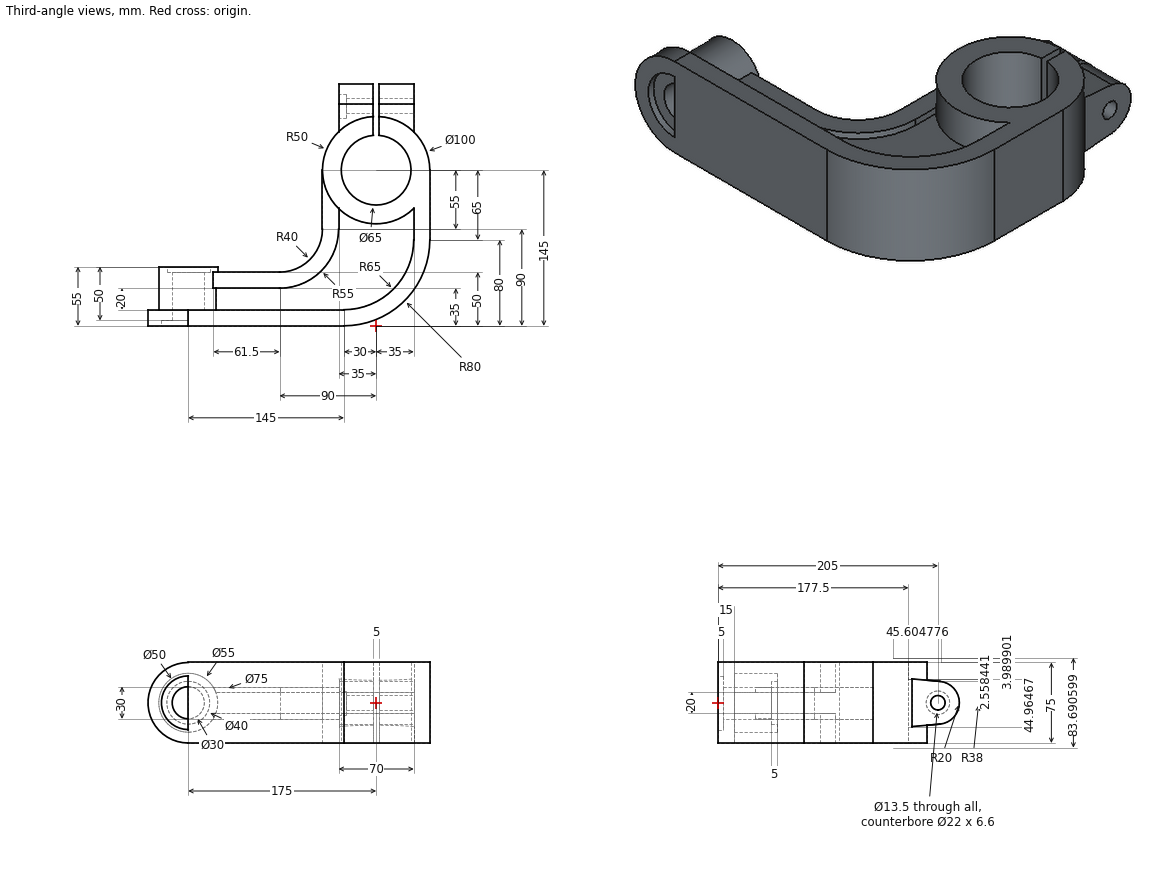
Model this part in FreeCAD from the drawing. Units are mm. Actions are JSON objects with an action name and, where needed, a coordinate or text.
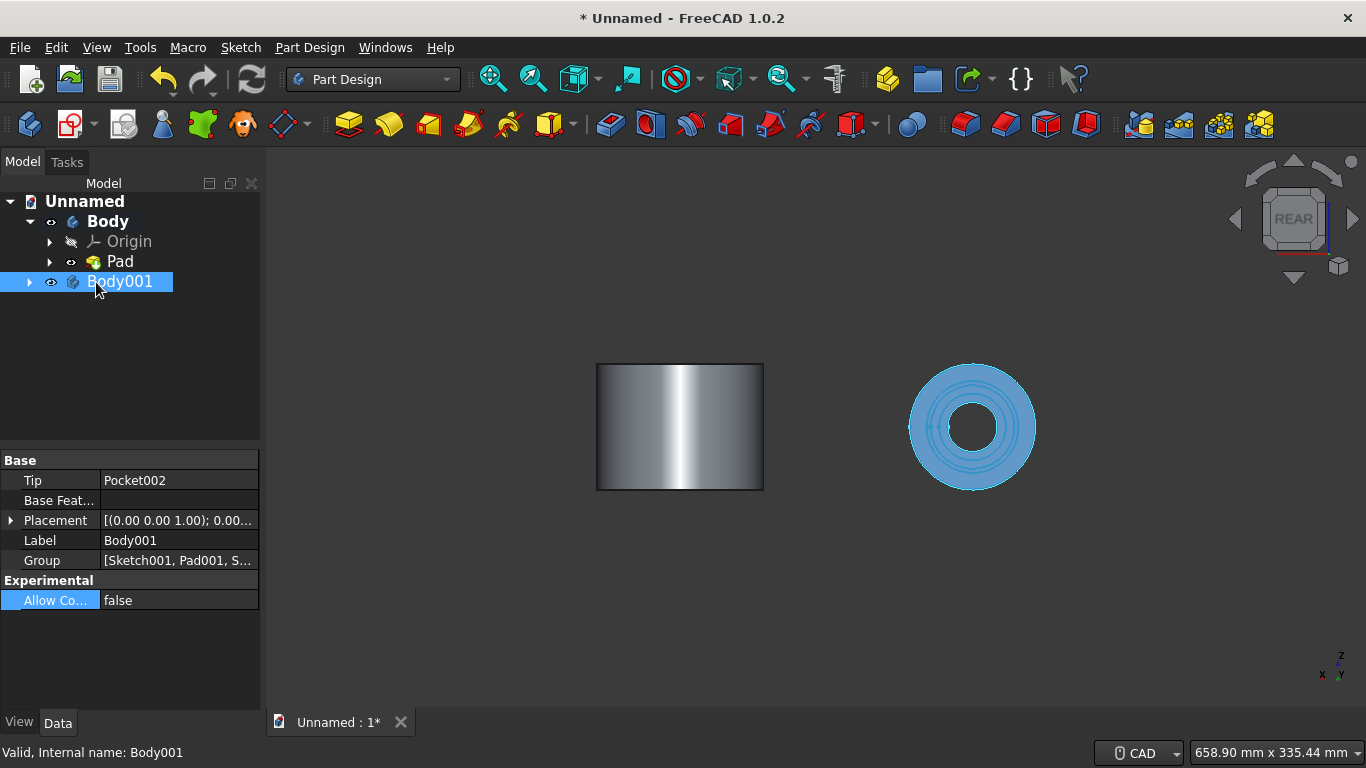
{"action": "left_click", "coordinate": [914, 124]}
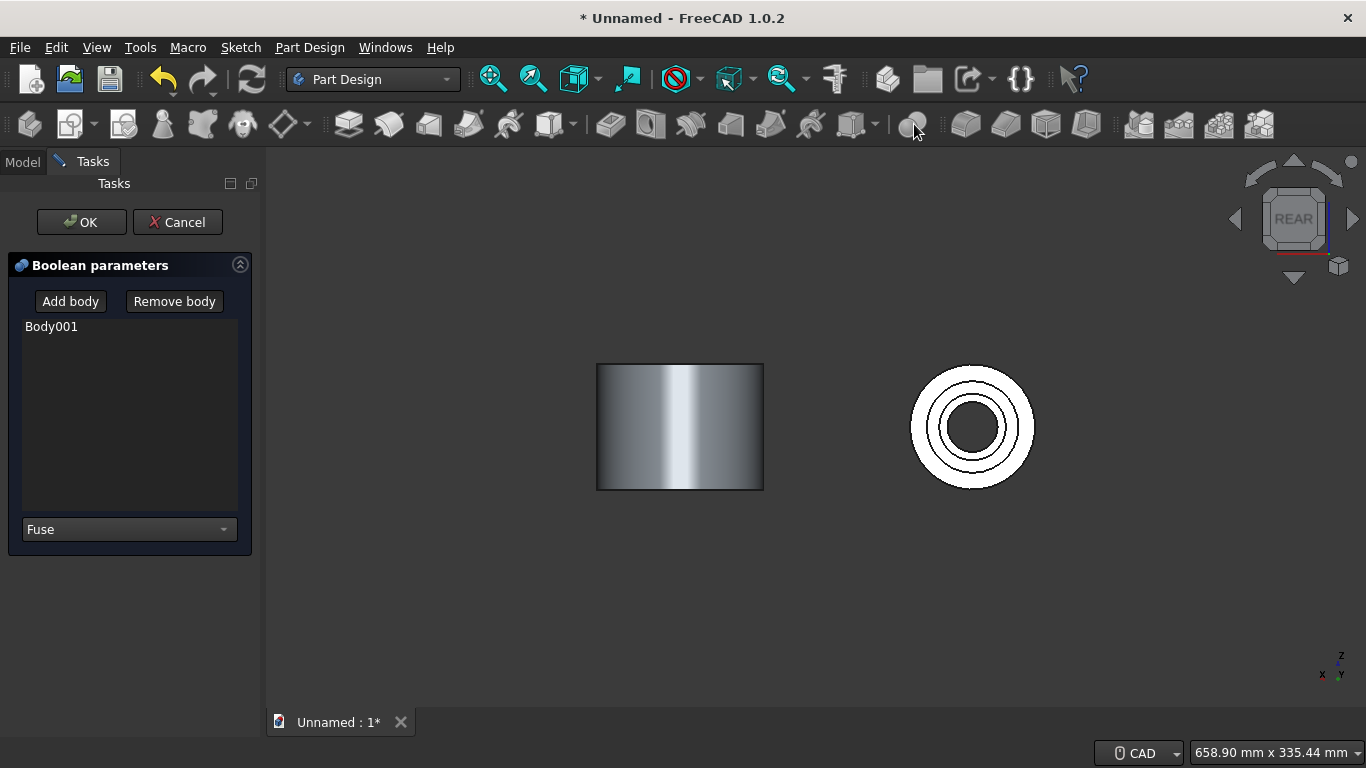
{"action": "left_click", "coordinate": [82, 222]}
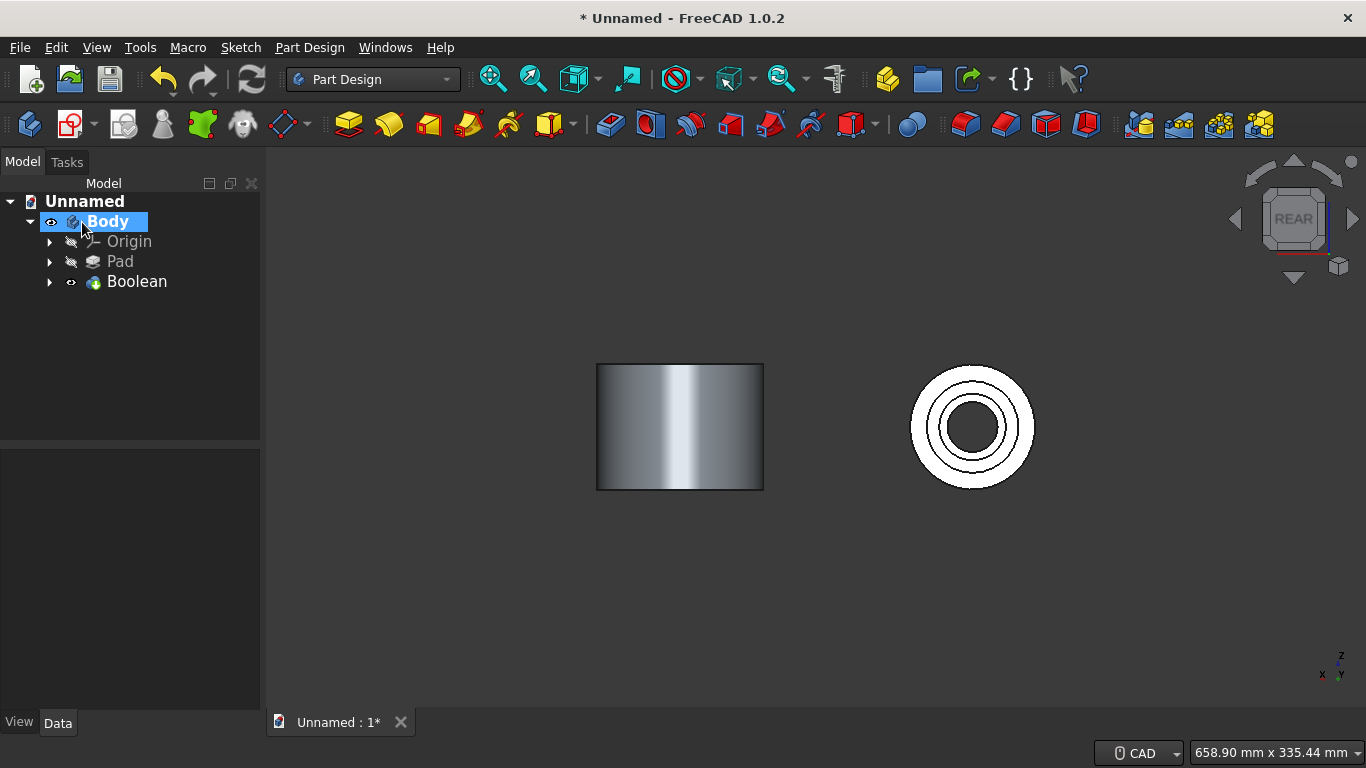
{"action": "key", "text": "v f"}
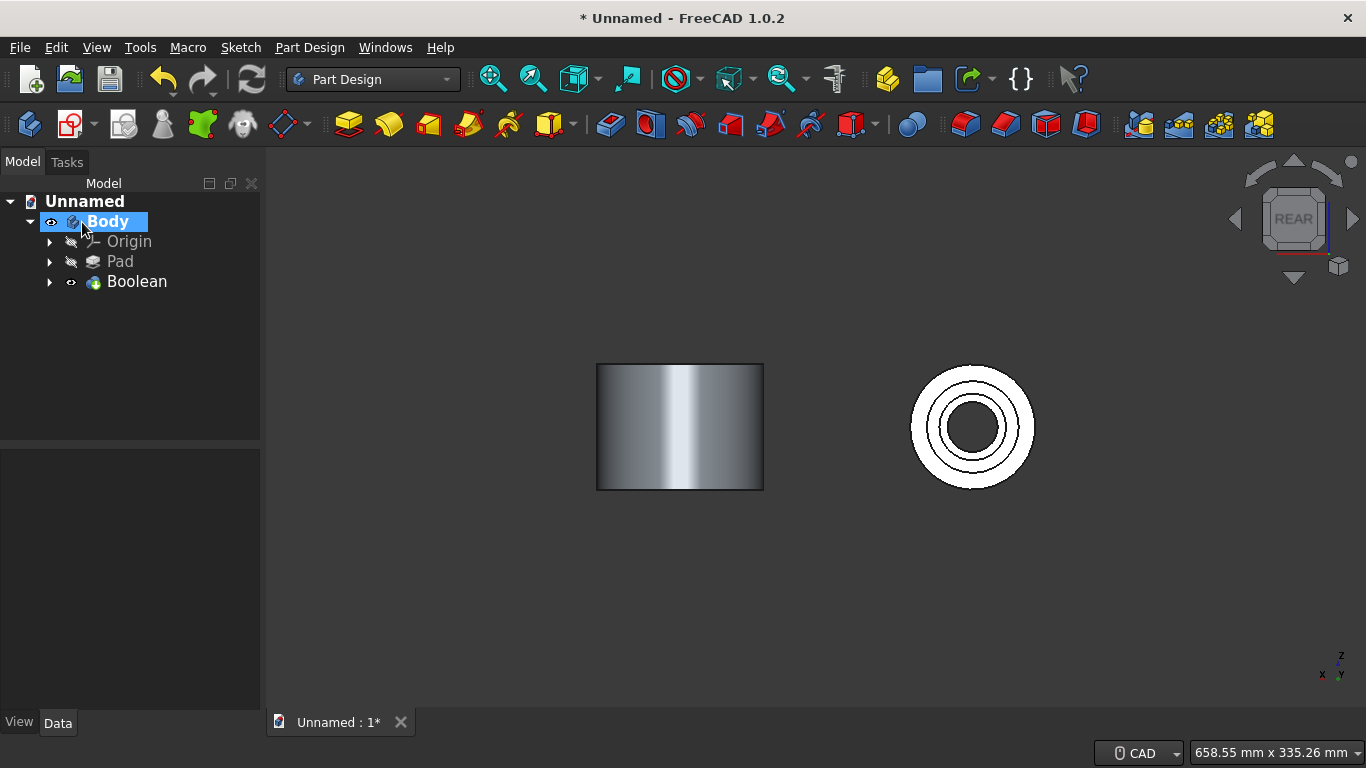
{"action": "left_click", "coordinate": [70, 124]}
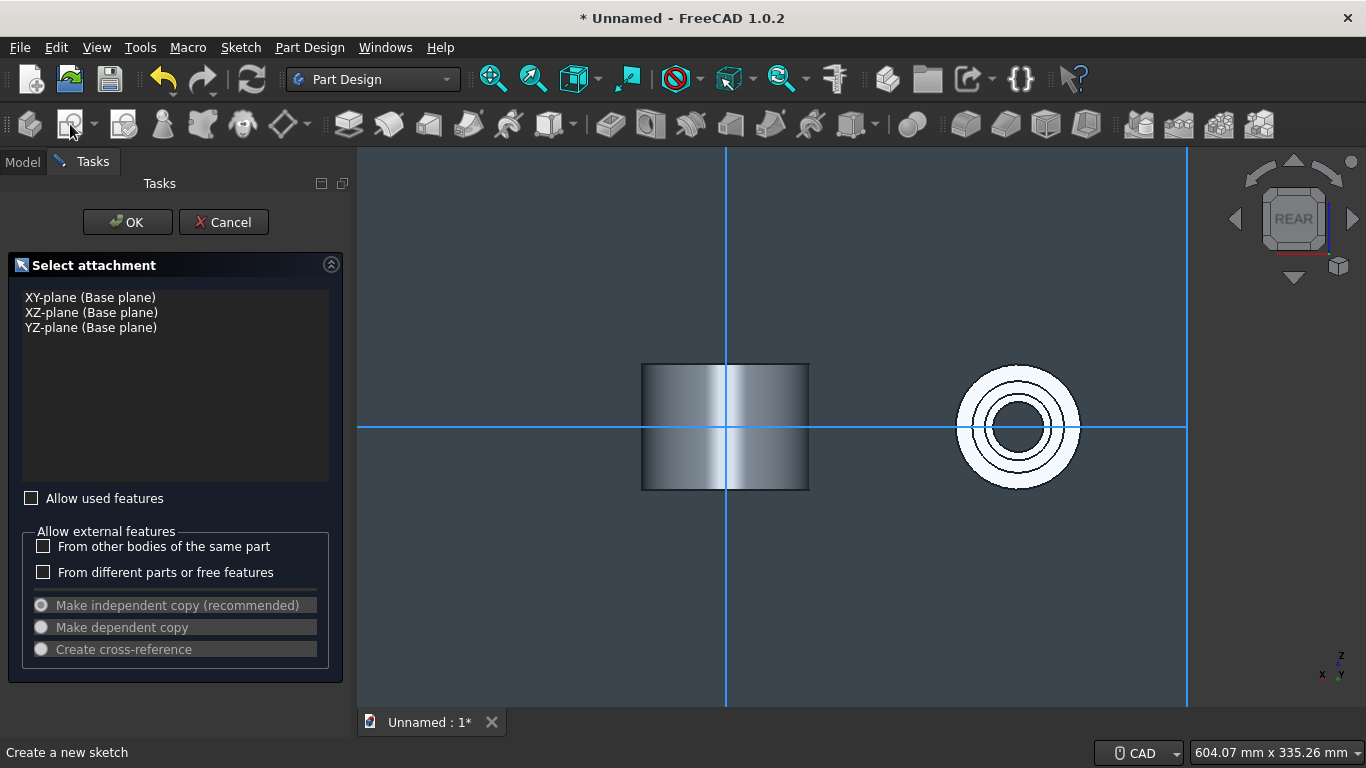
{"action": "left_click", "coordinate": [82, 298]}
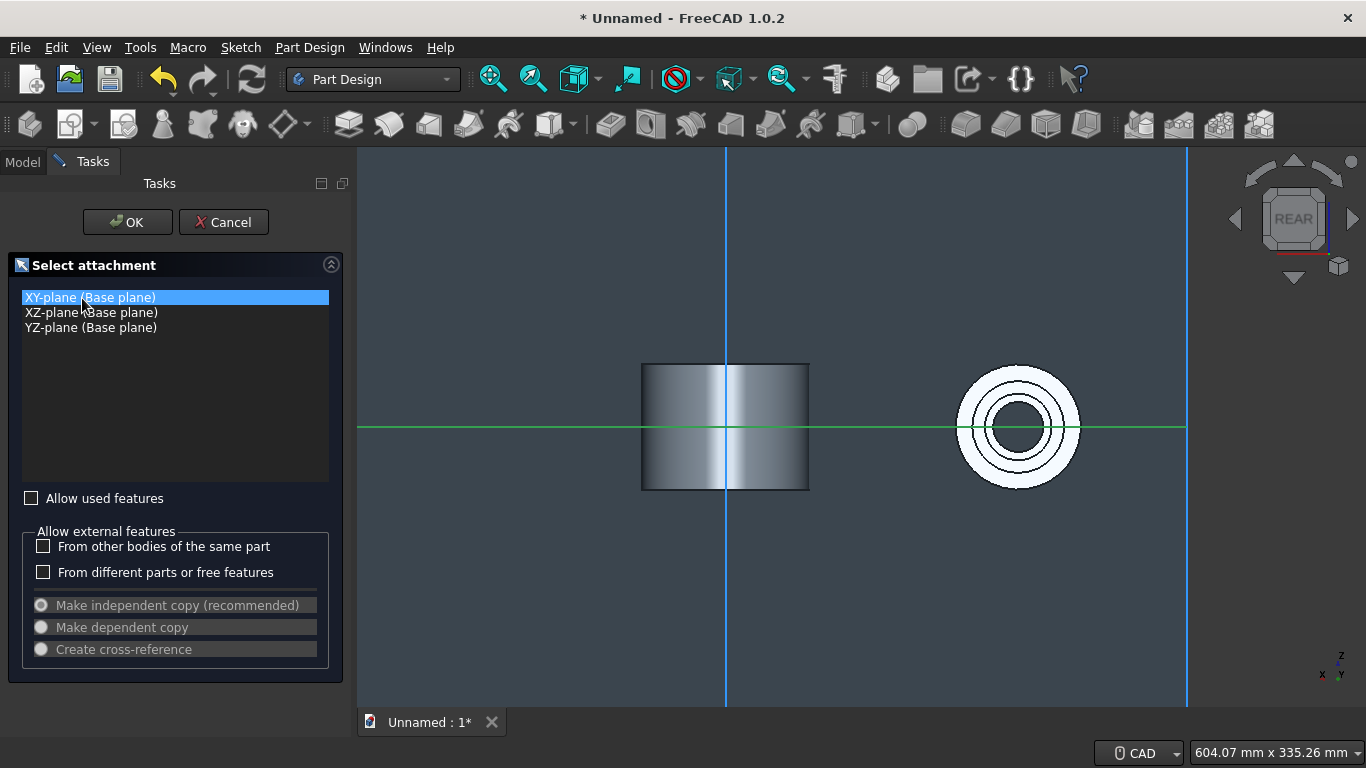
{"action": "left_click", "coordinate": [128, 222]}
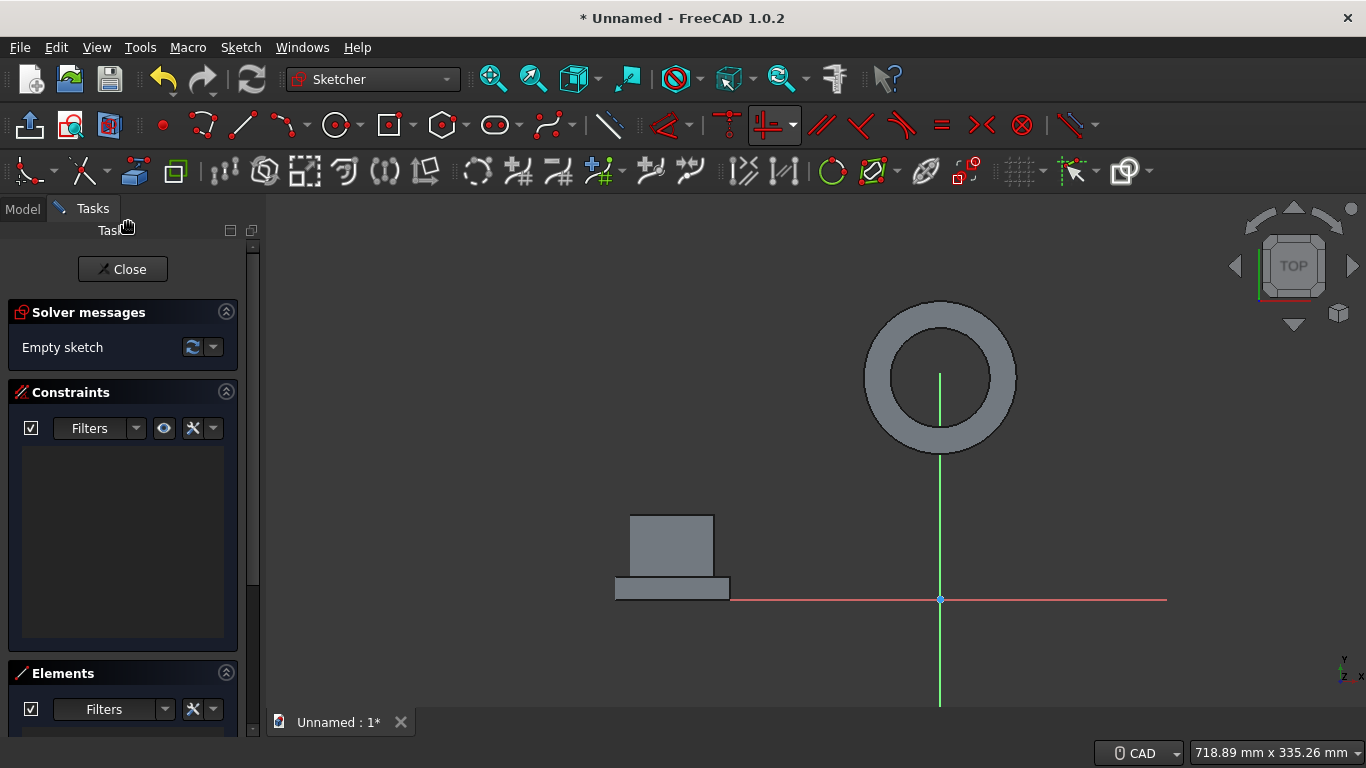
{"action": "left_click", "coordinate": [110, 126]}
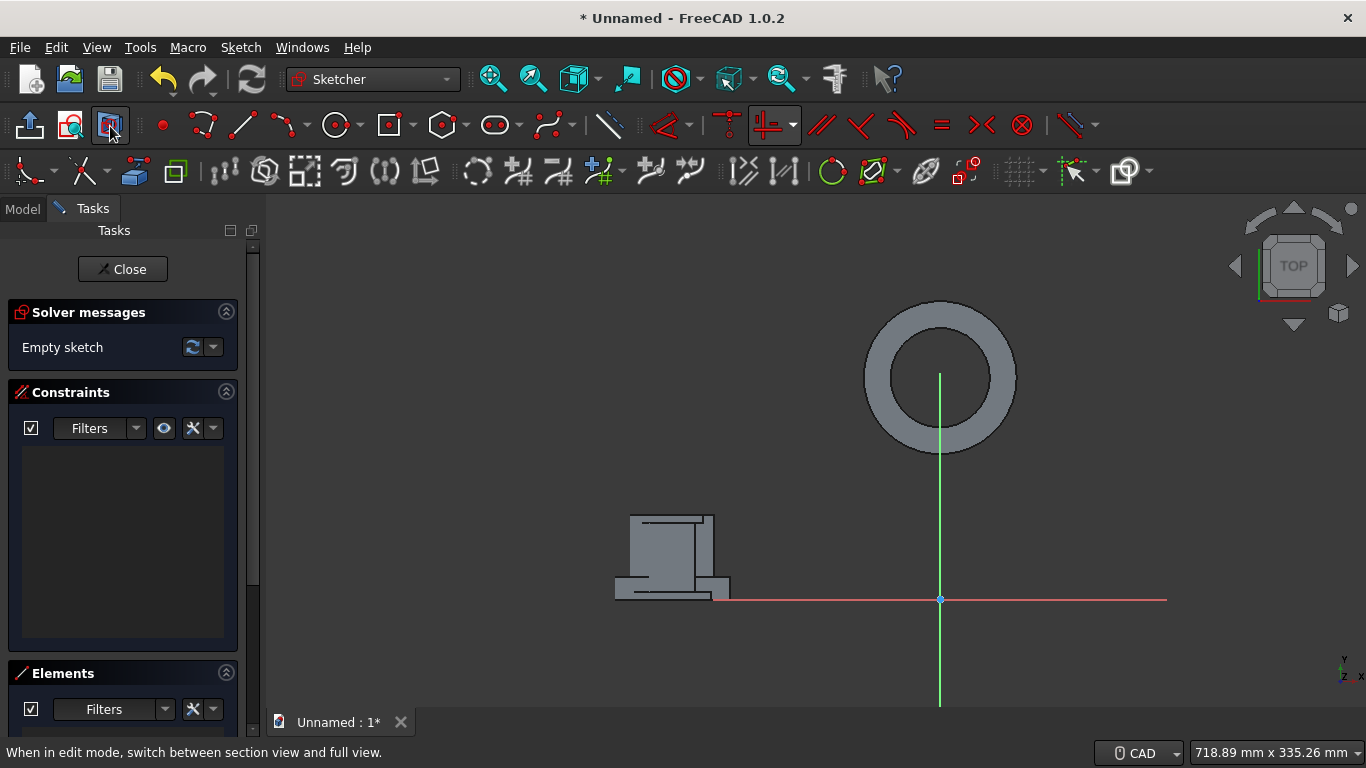
{"action": "key", "text": "g l"}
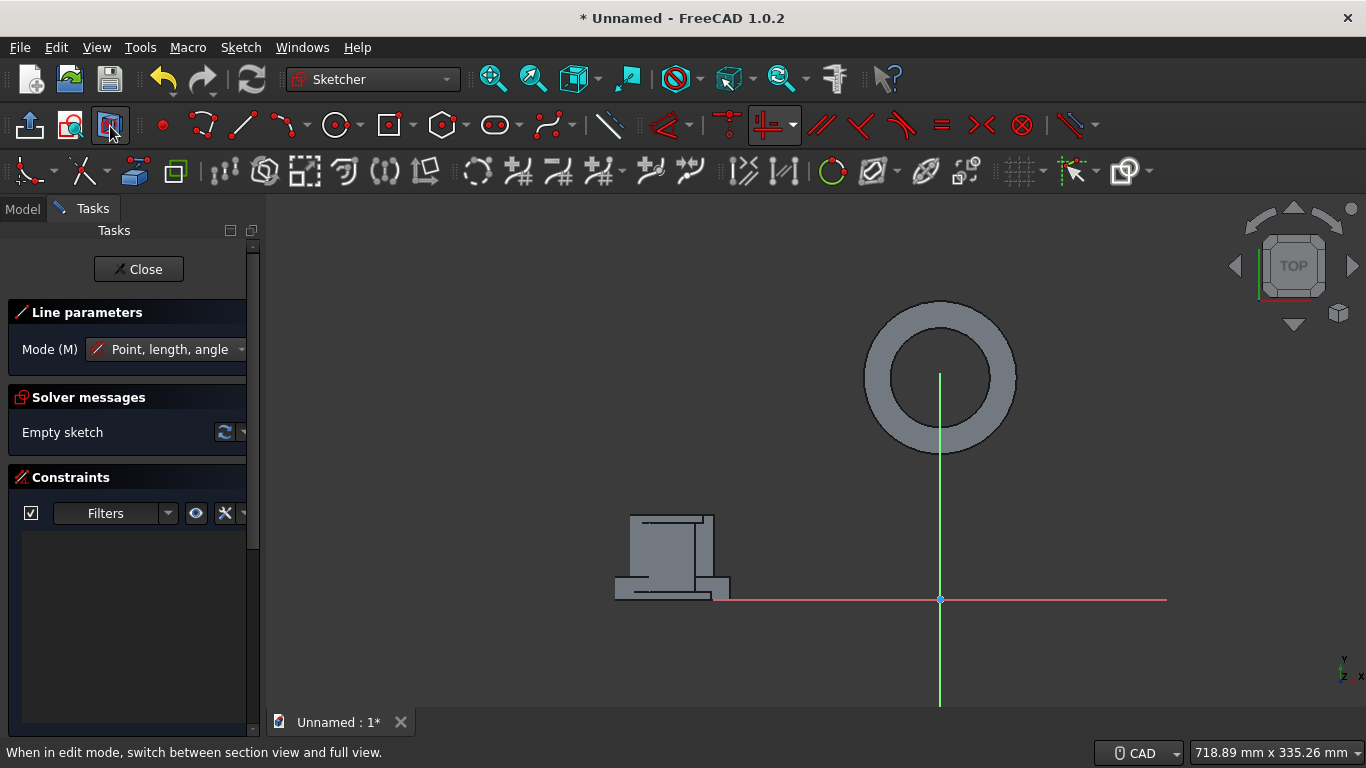
{"action": "left_click", "coordinate": [1017, 477]}
{"action": "left_click", "coordinate": [1017, 378]}